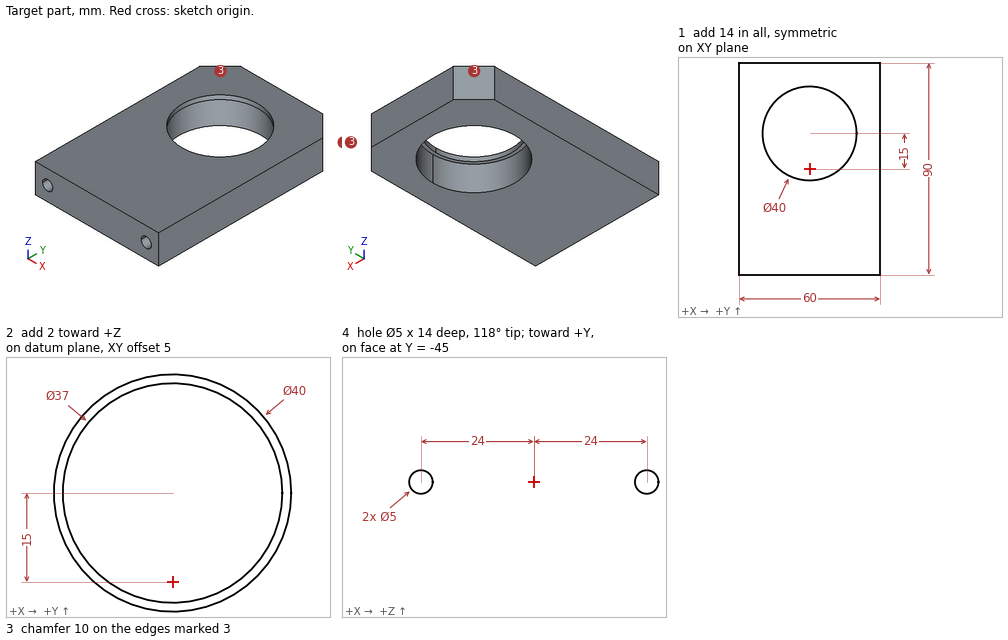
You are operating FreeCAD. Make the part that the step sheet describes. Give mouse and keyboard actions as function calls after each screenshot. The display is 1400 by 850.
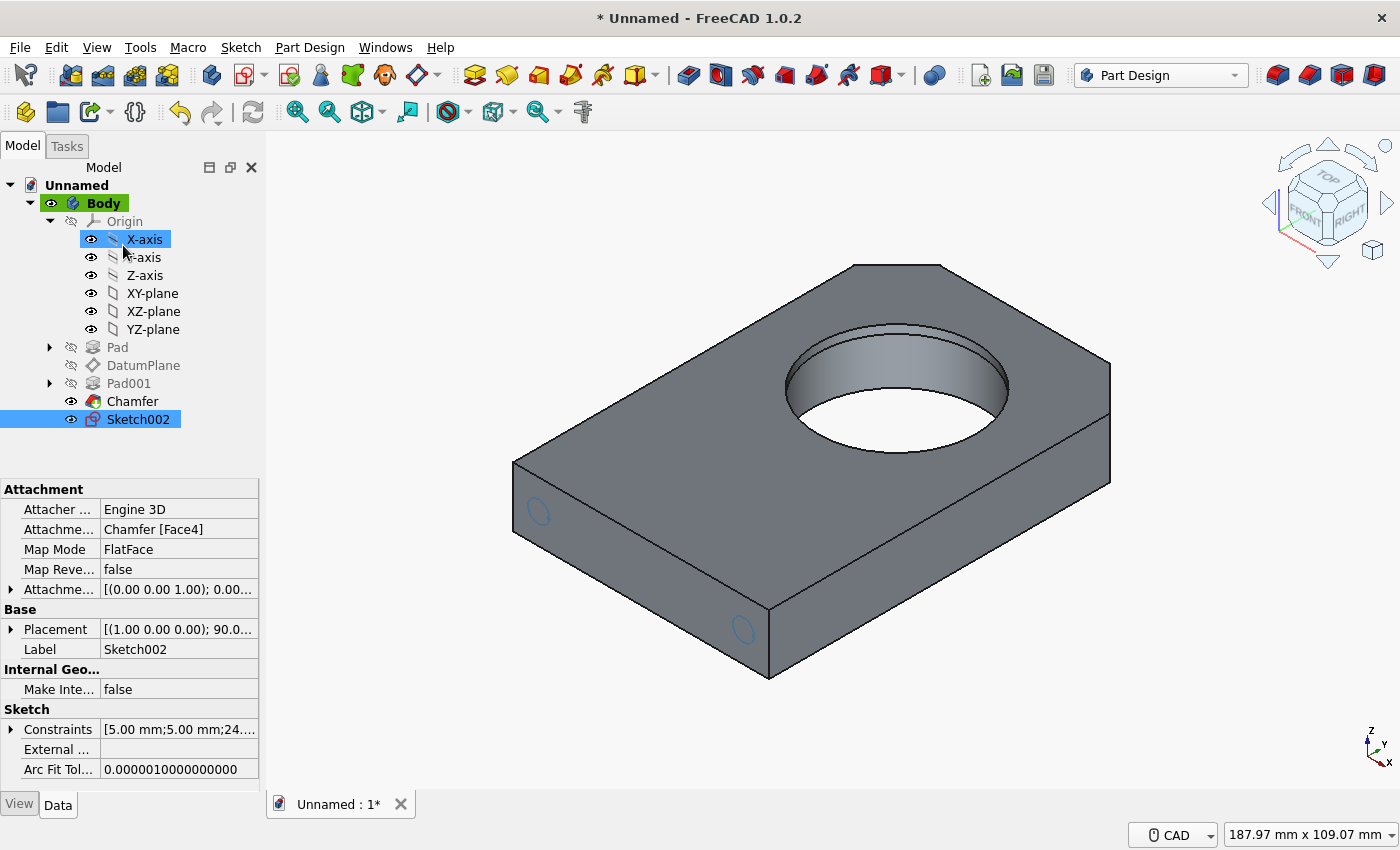
click(722, 76)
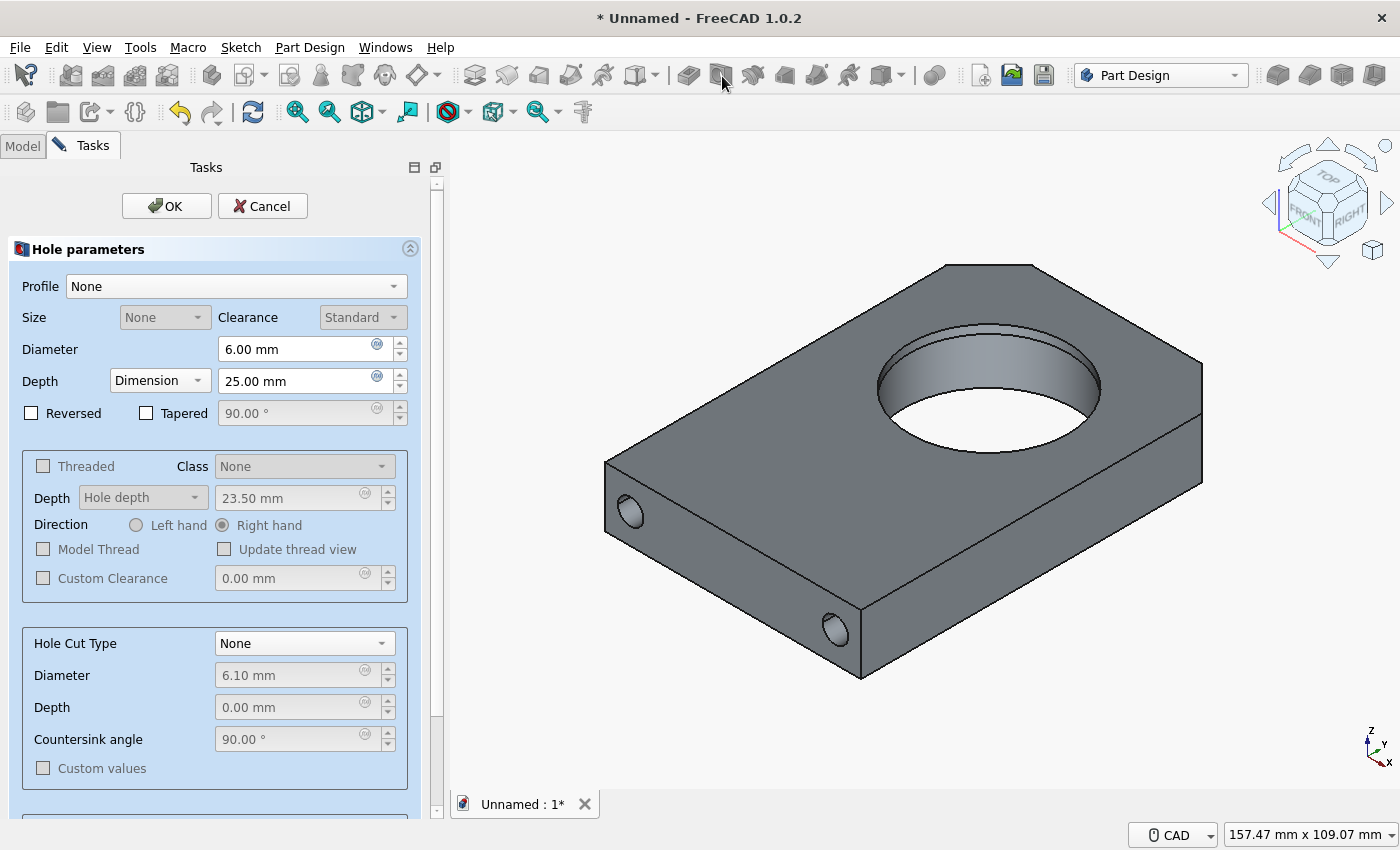
triple_click(305, 349)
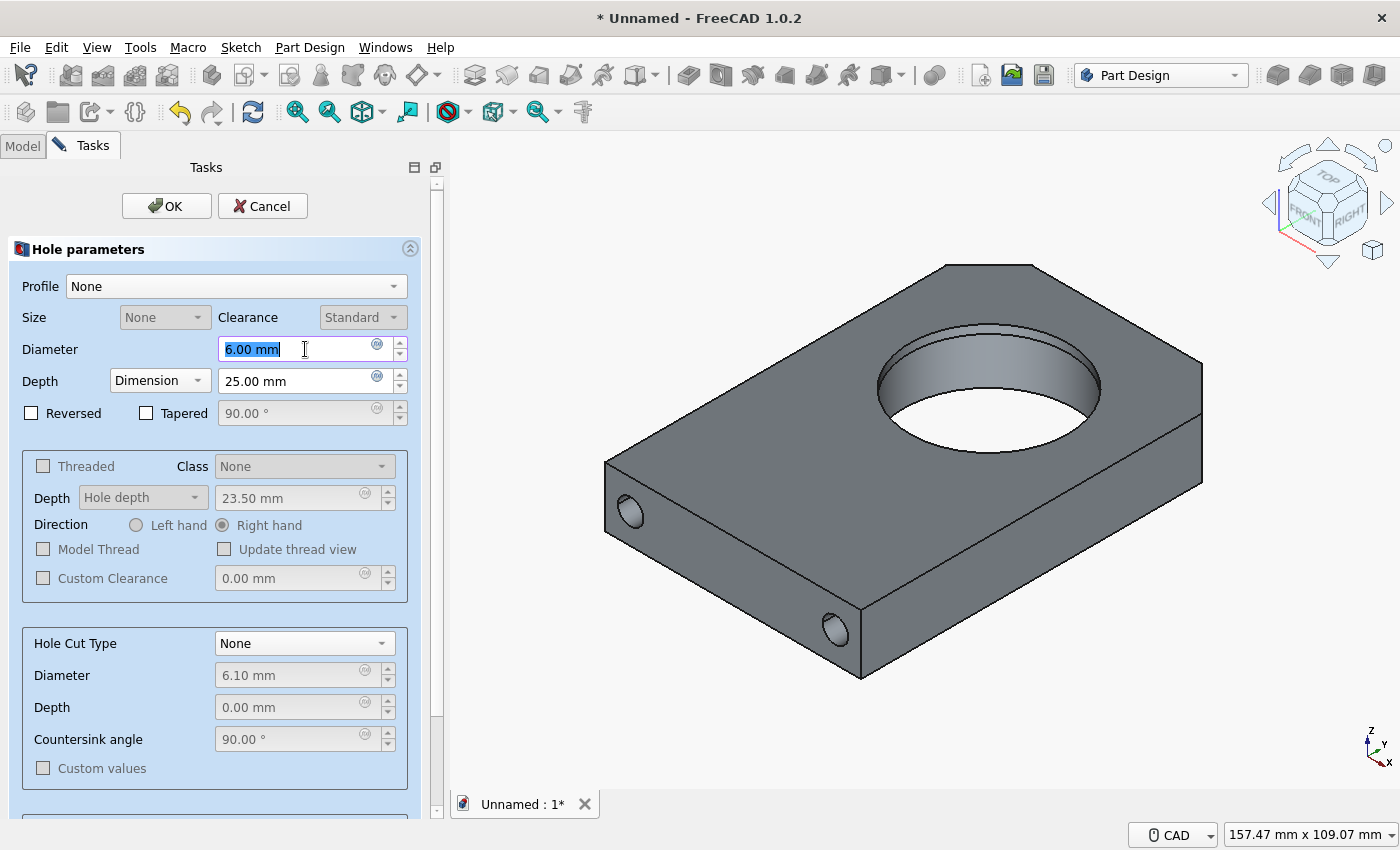
text(5)
key(Tab)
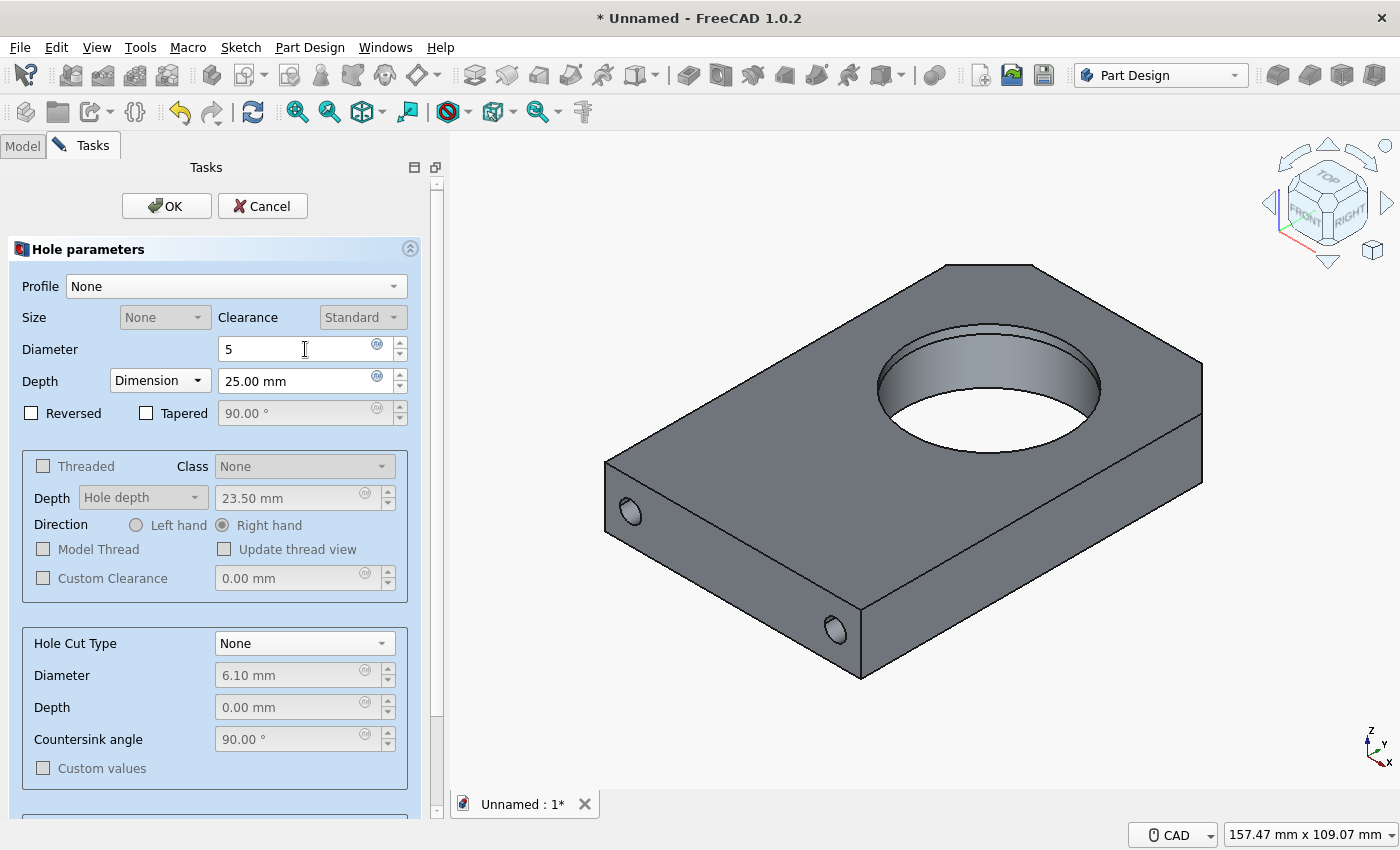
triple_click(305, 381)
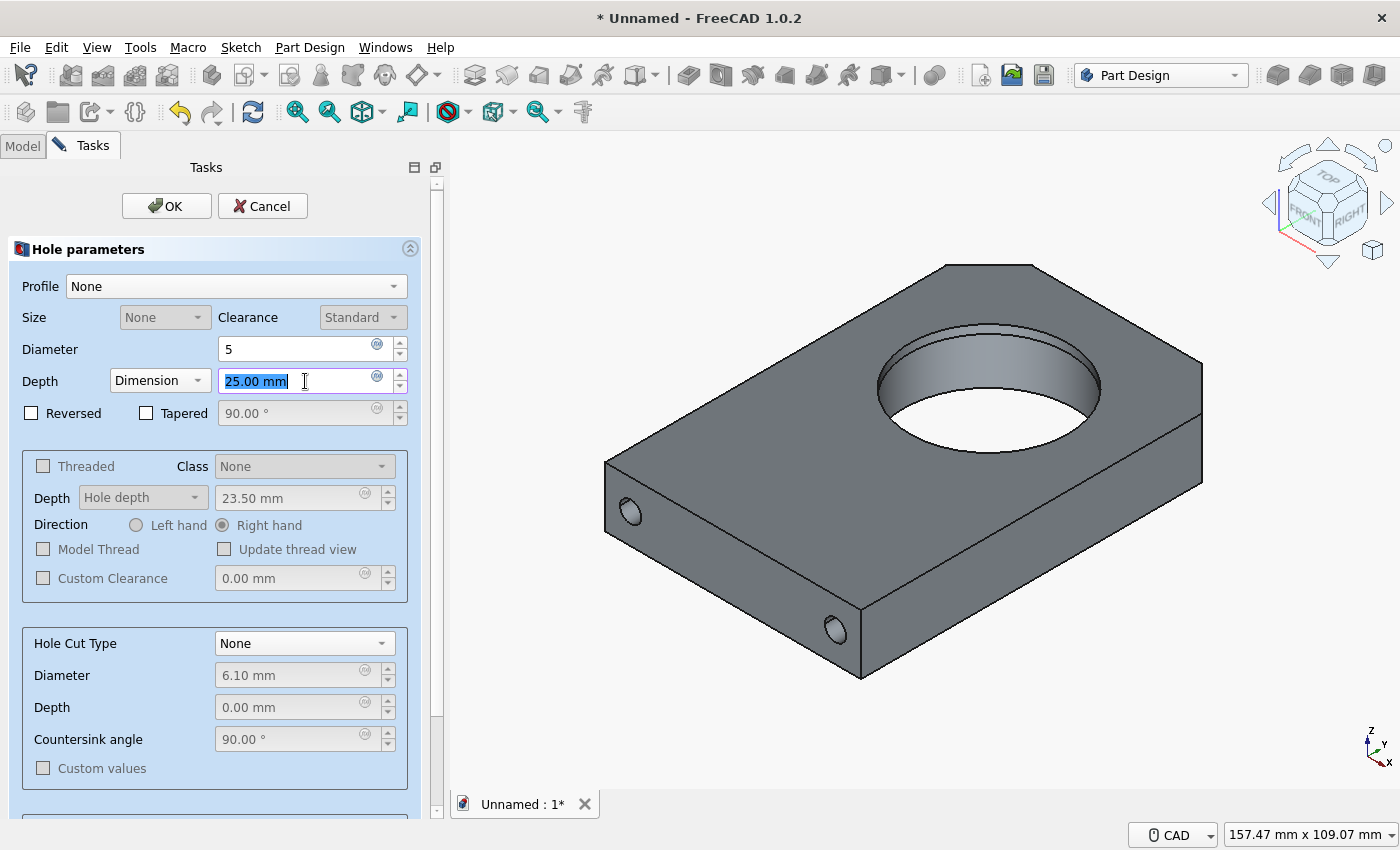
text(14)
key(Tab)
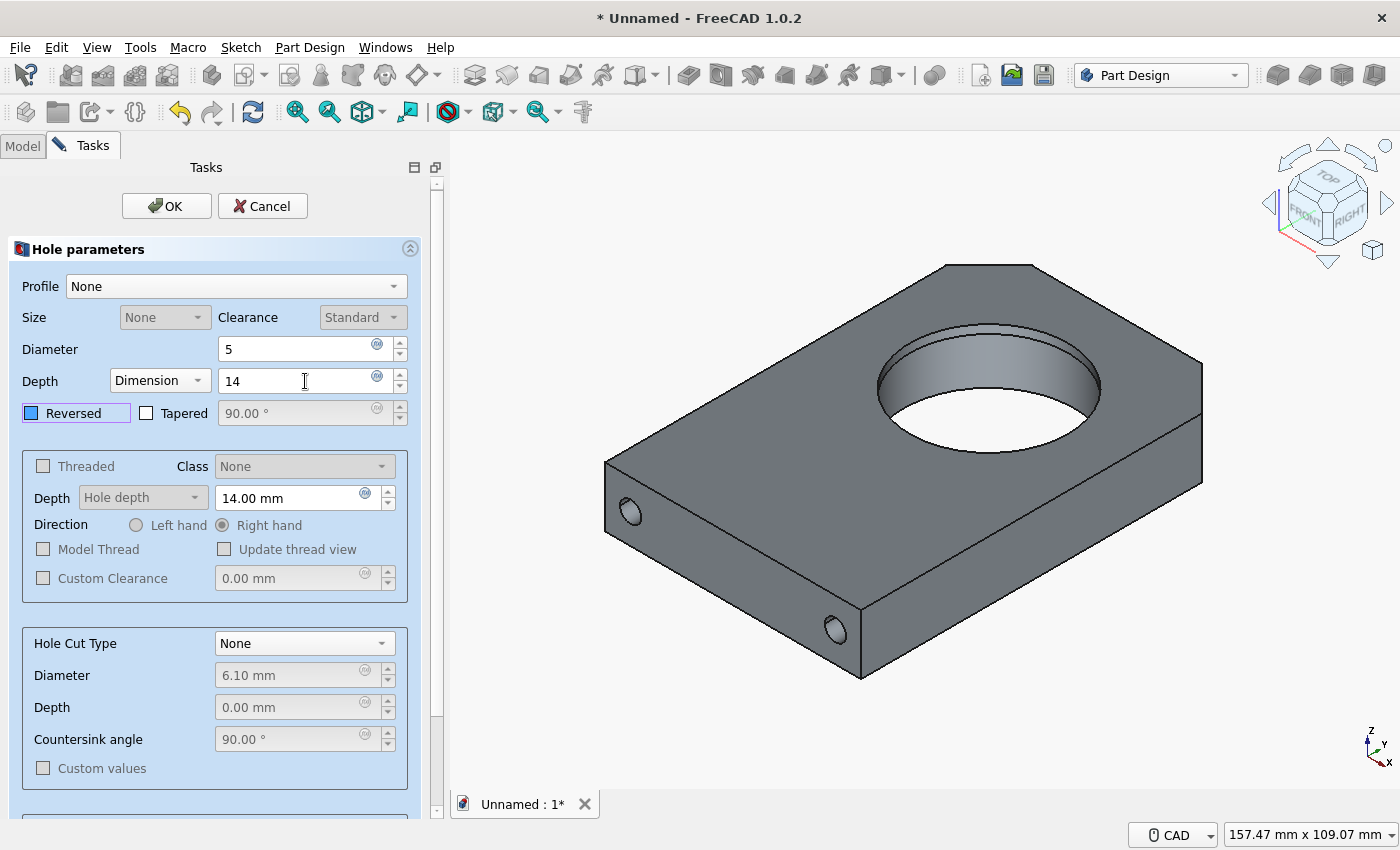
click(167, 206)